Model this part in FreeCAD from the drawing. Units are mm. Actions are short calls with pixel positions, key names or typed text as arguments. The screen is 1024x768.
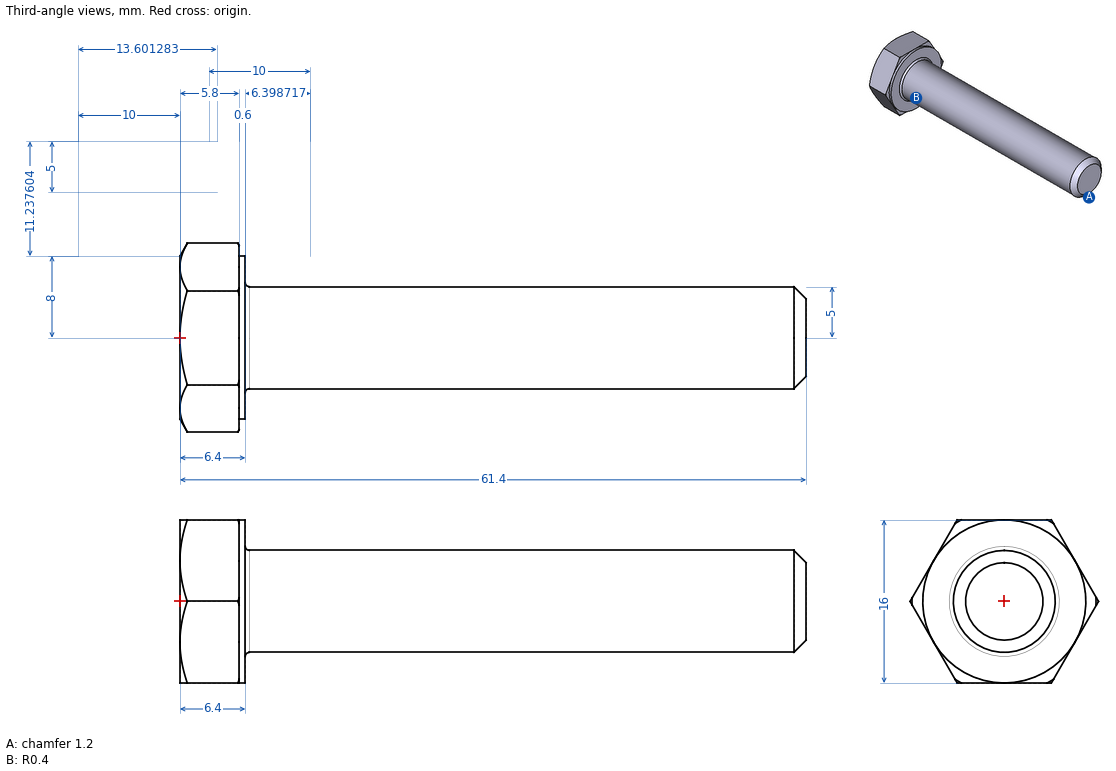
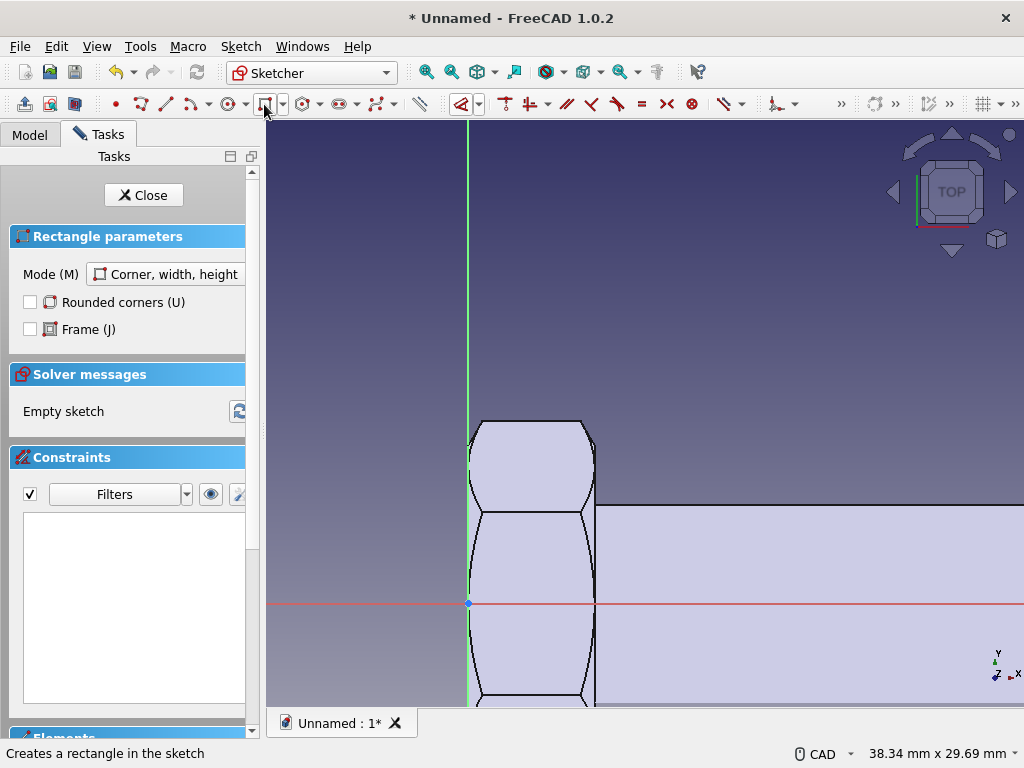
scroll(583, 223, up, 2)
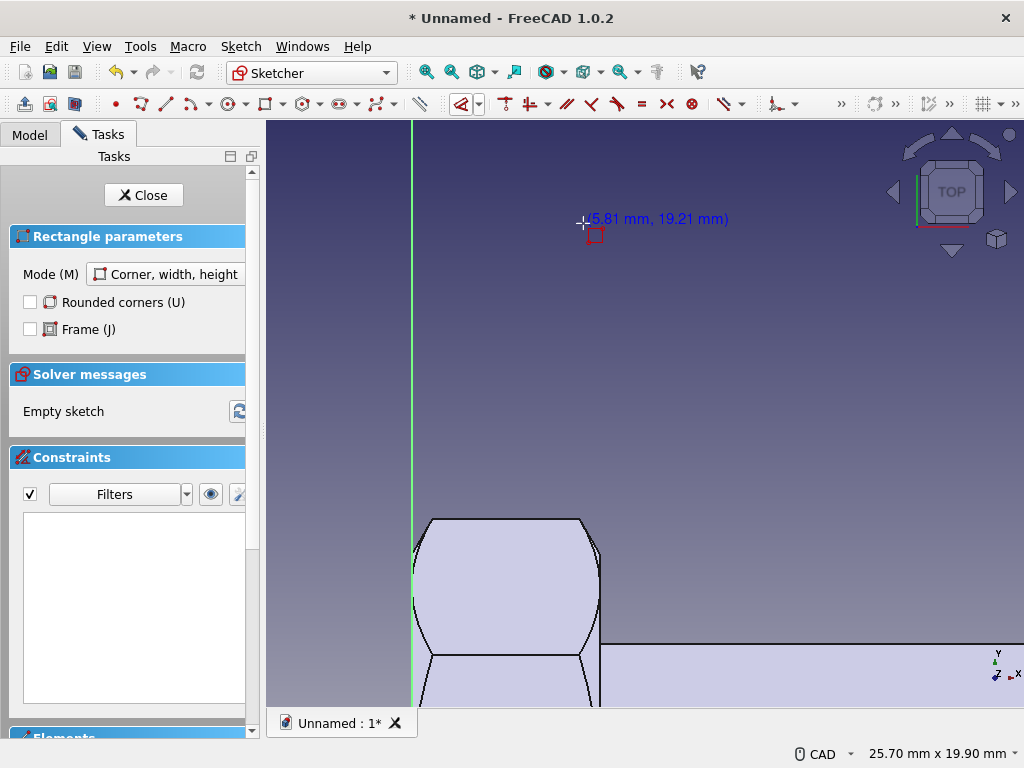
click(583, 224)
move(600, 555)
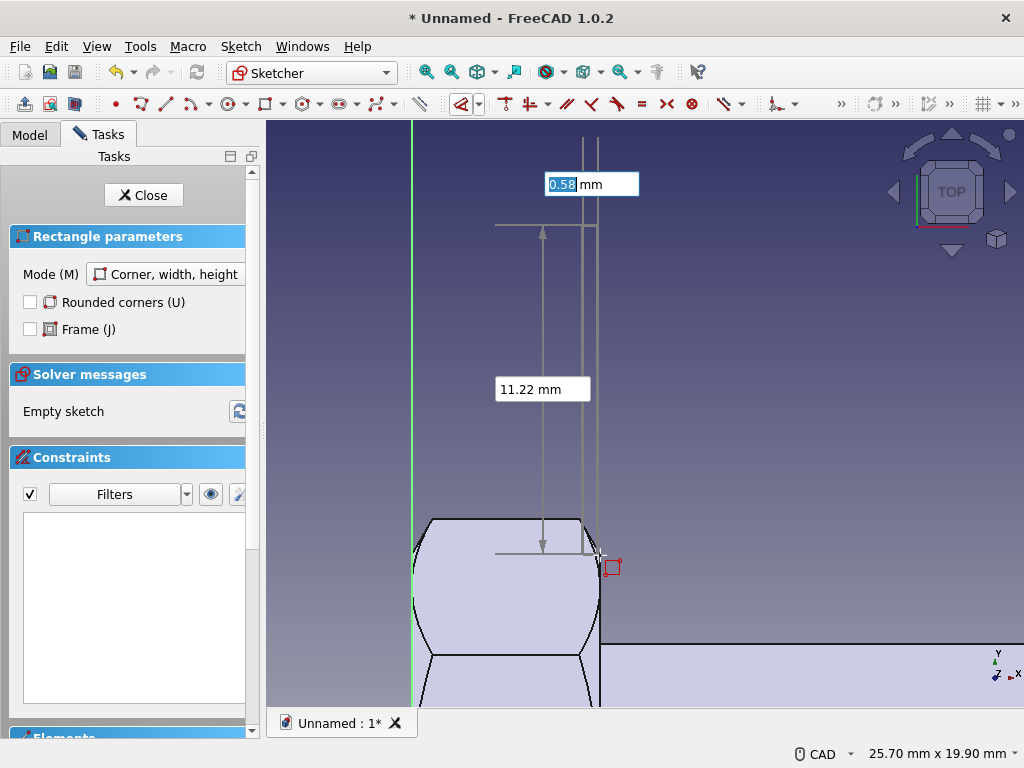
text(0.6)
key(Tab)
text(11.237604)
key(Return)
key(Escape)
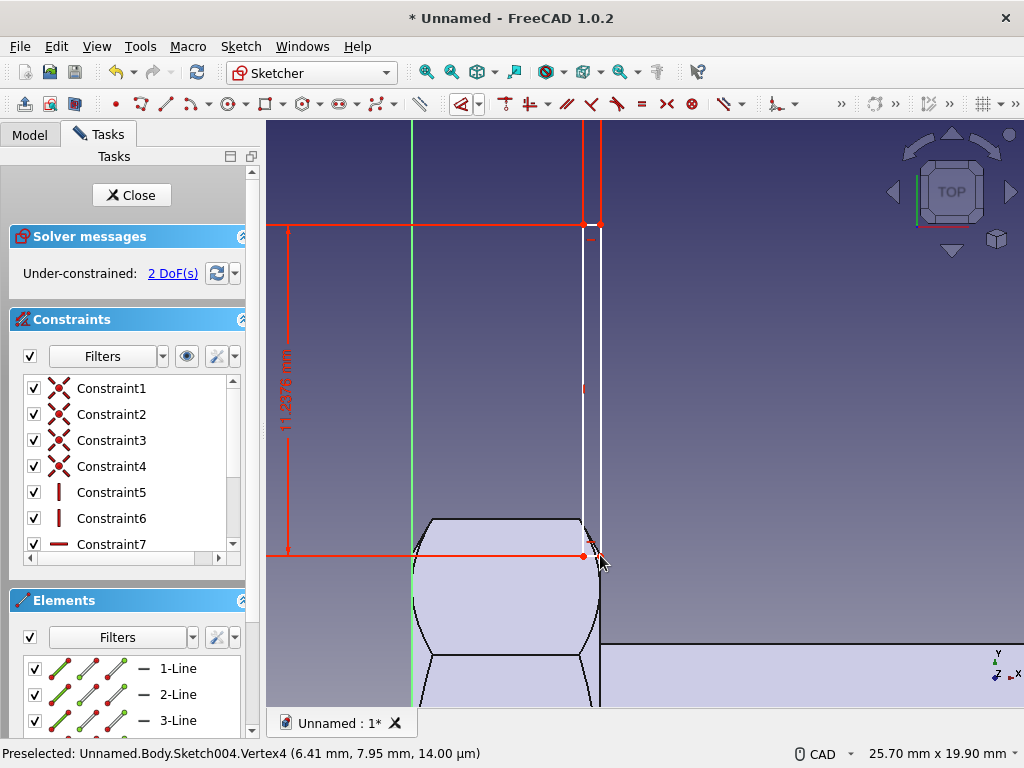
click(583, 556)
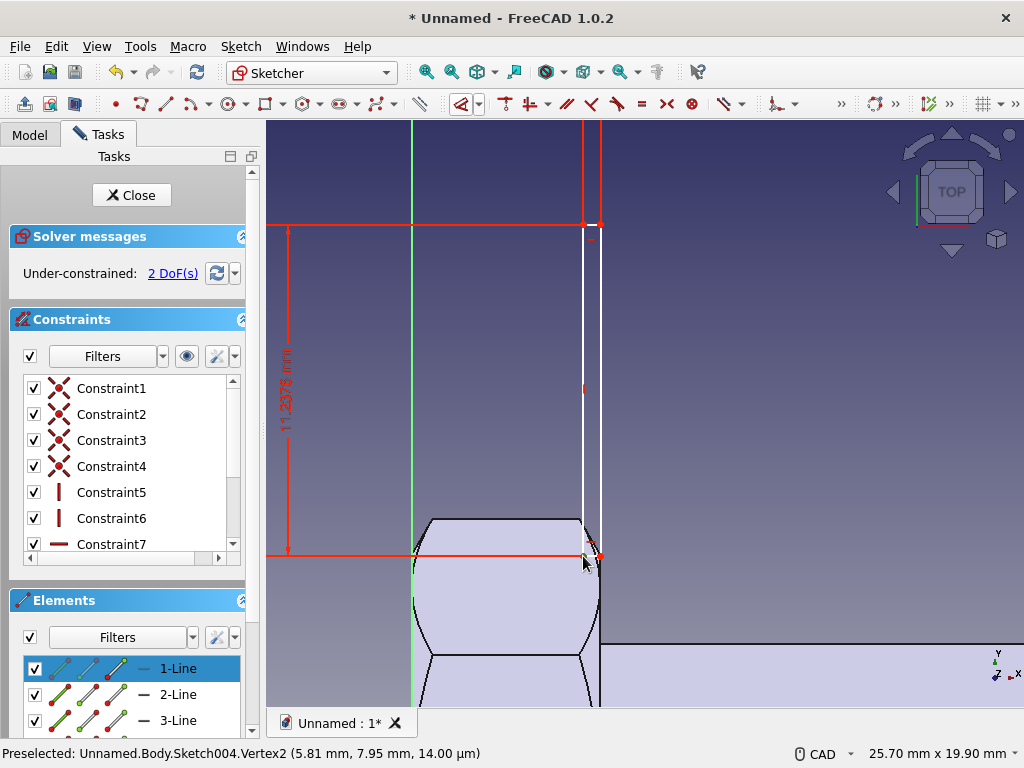
click(478, 104)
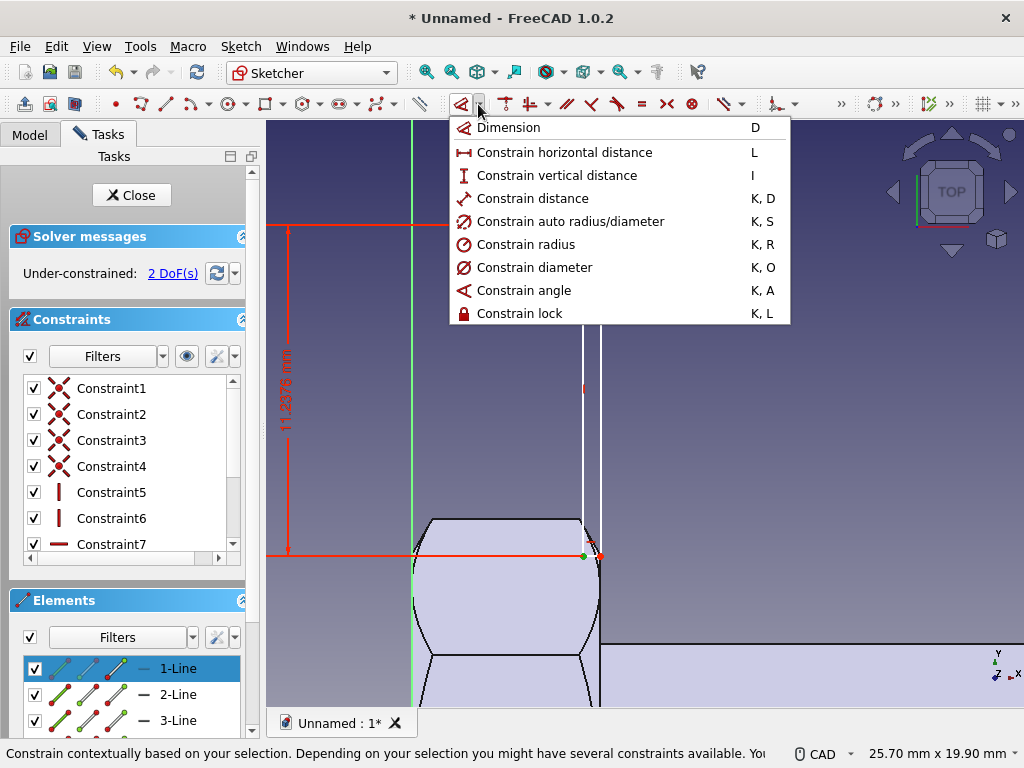
click(620, 176)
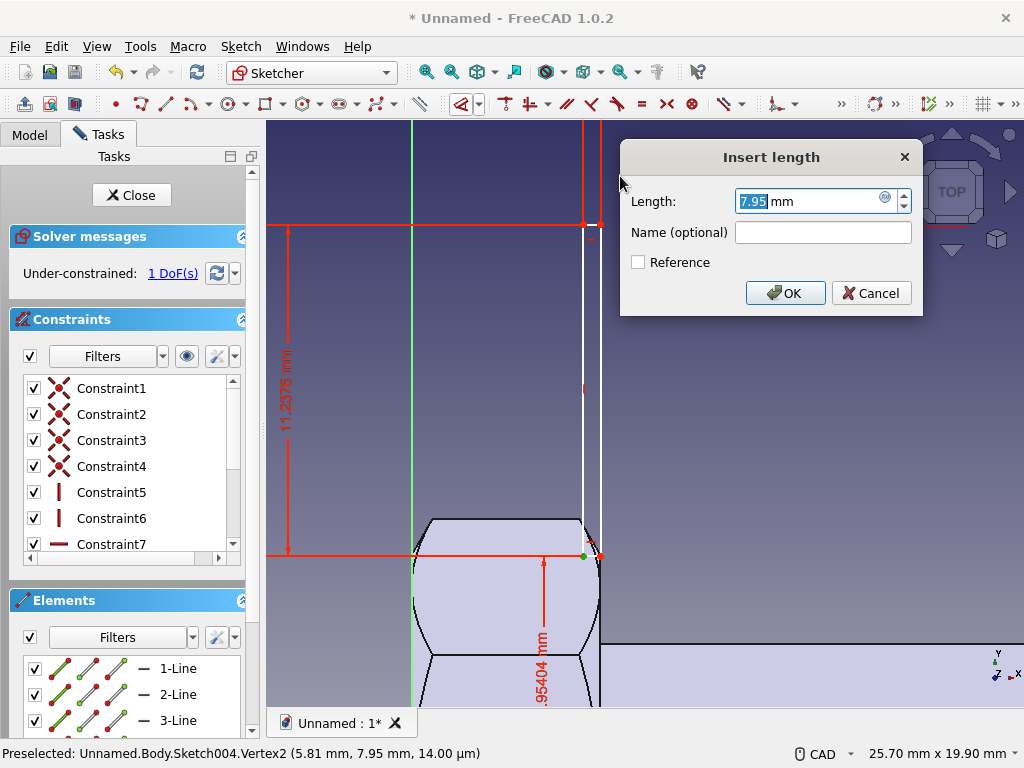
text(8)
key(Return)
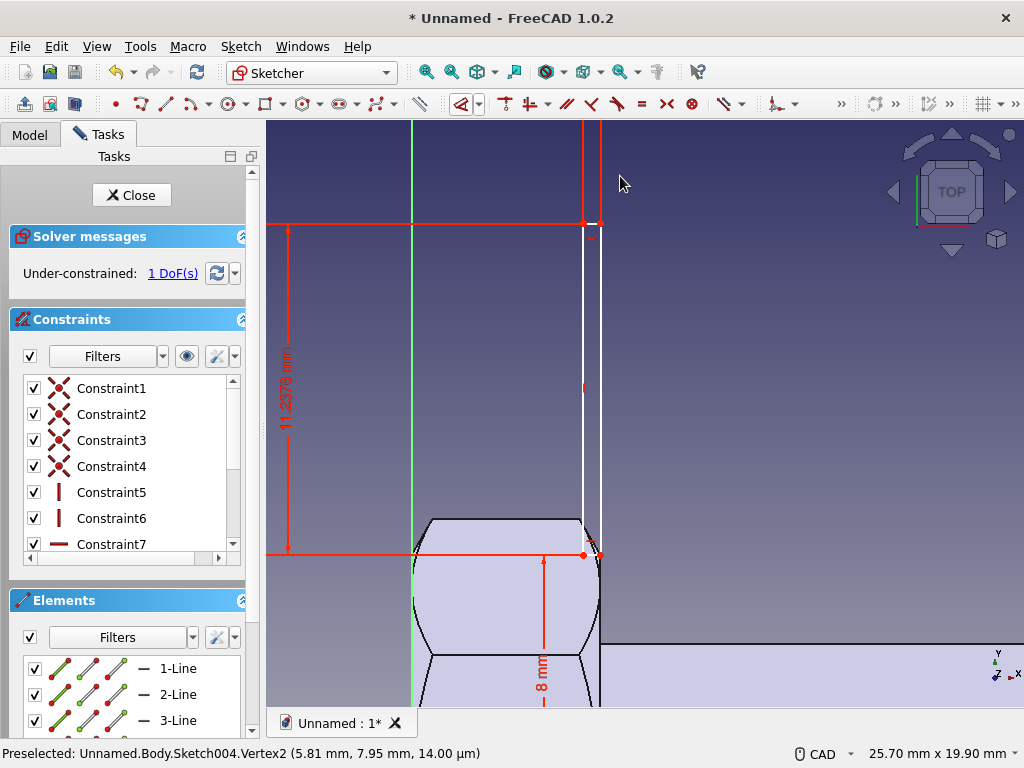
click(583, 224)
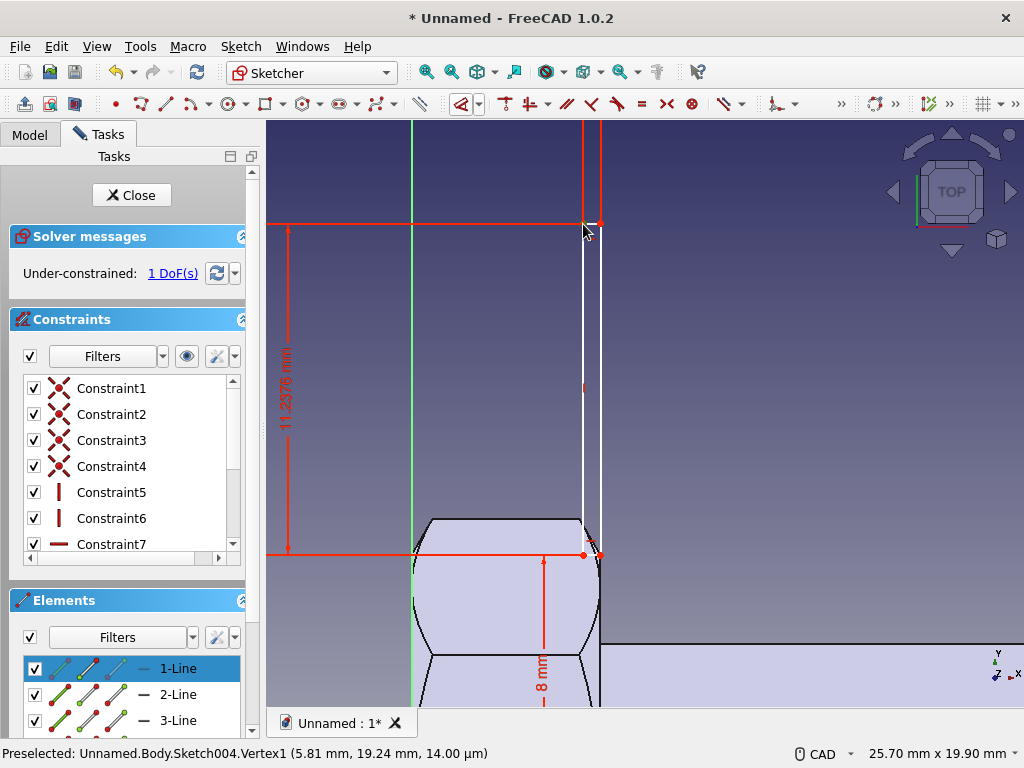
click(478, 104)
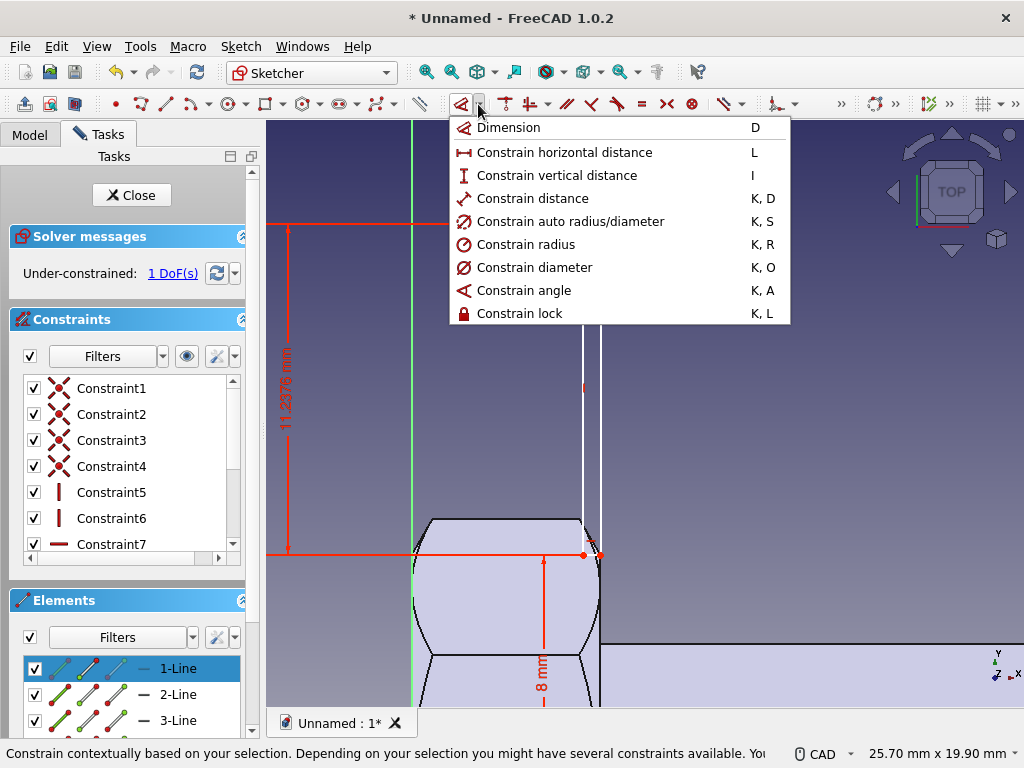
click(620, 152)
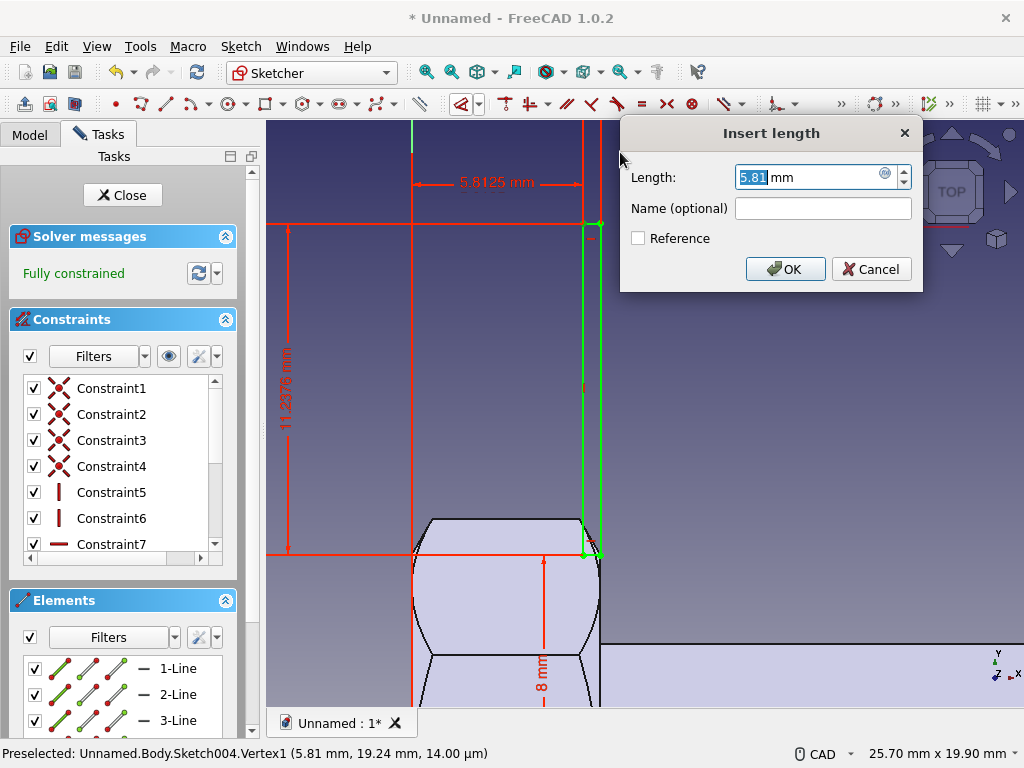
text(5.8)
key(Return)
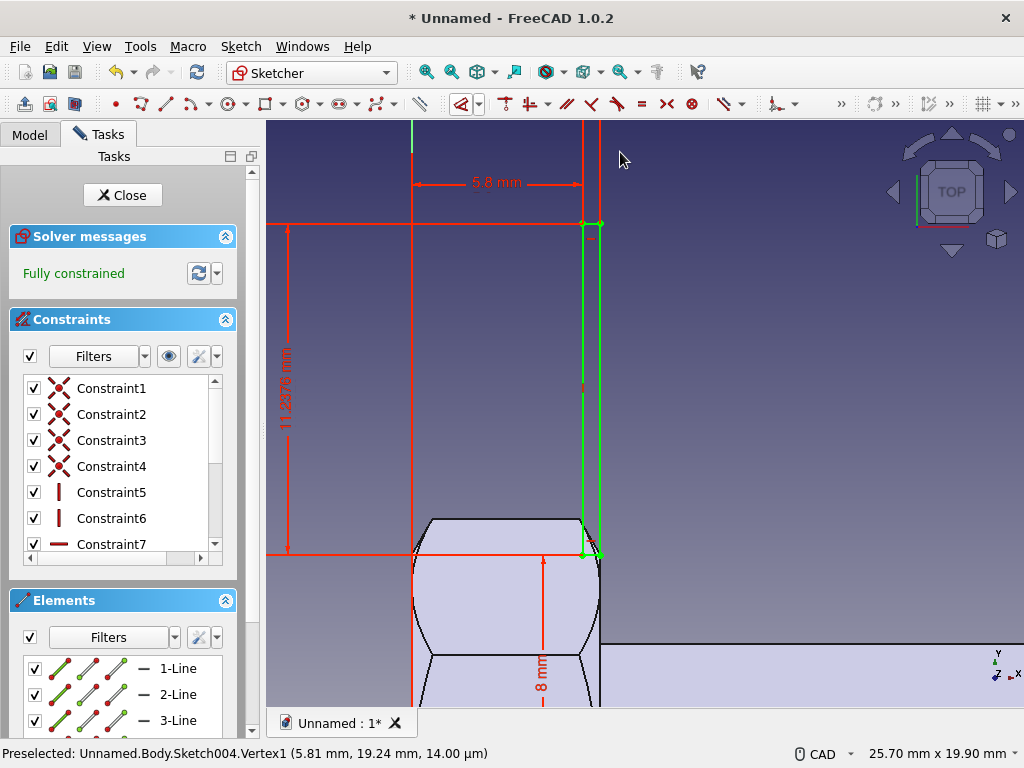
click(123, 195)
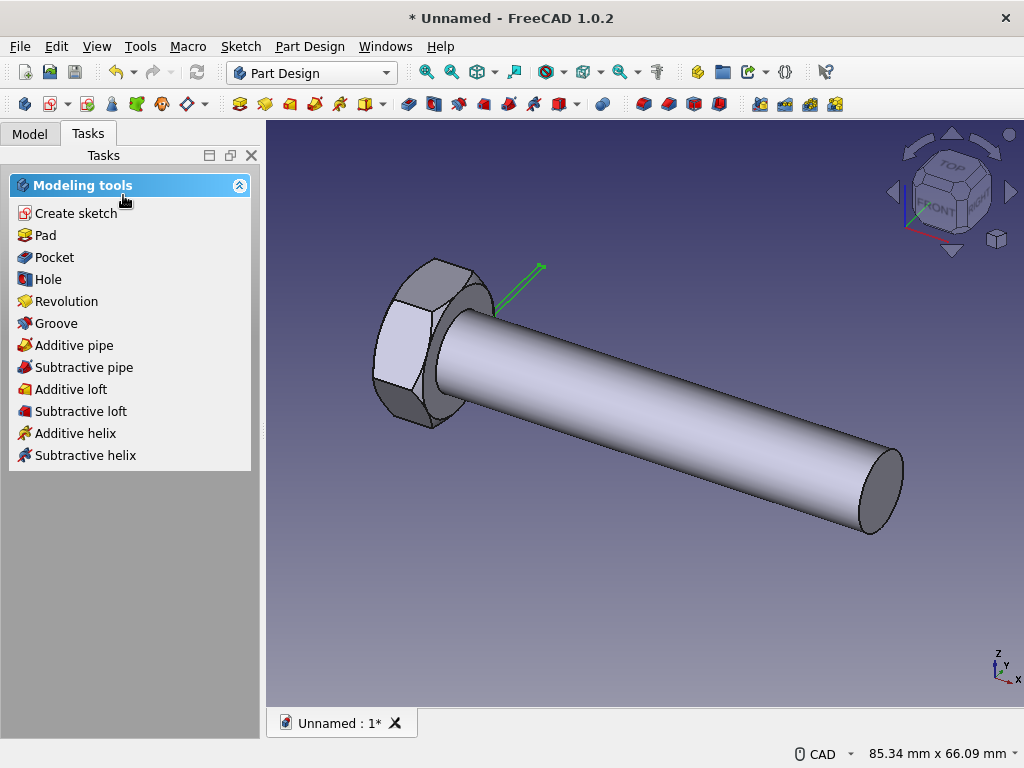
click(459, 104)